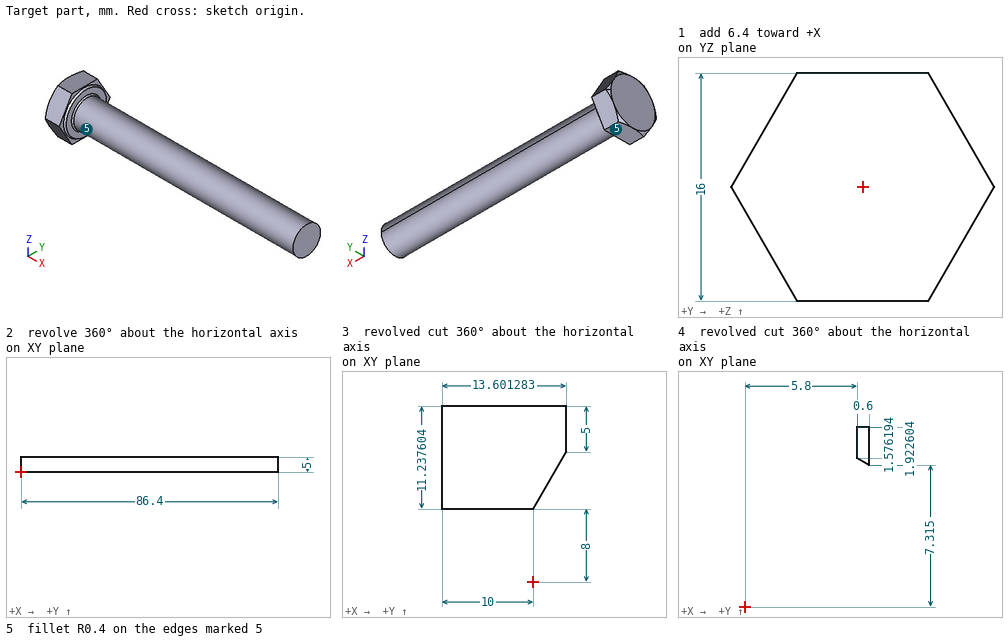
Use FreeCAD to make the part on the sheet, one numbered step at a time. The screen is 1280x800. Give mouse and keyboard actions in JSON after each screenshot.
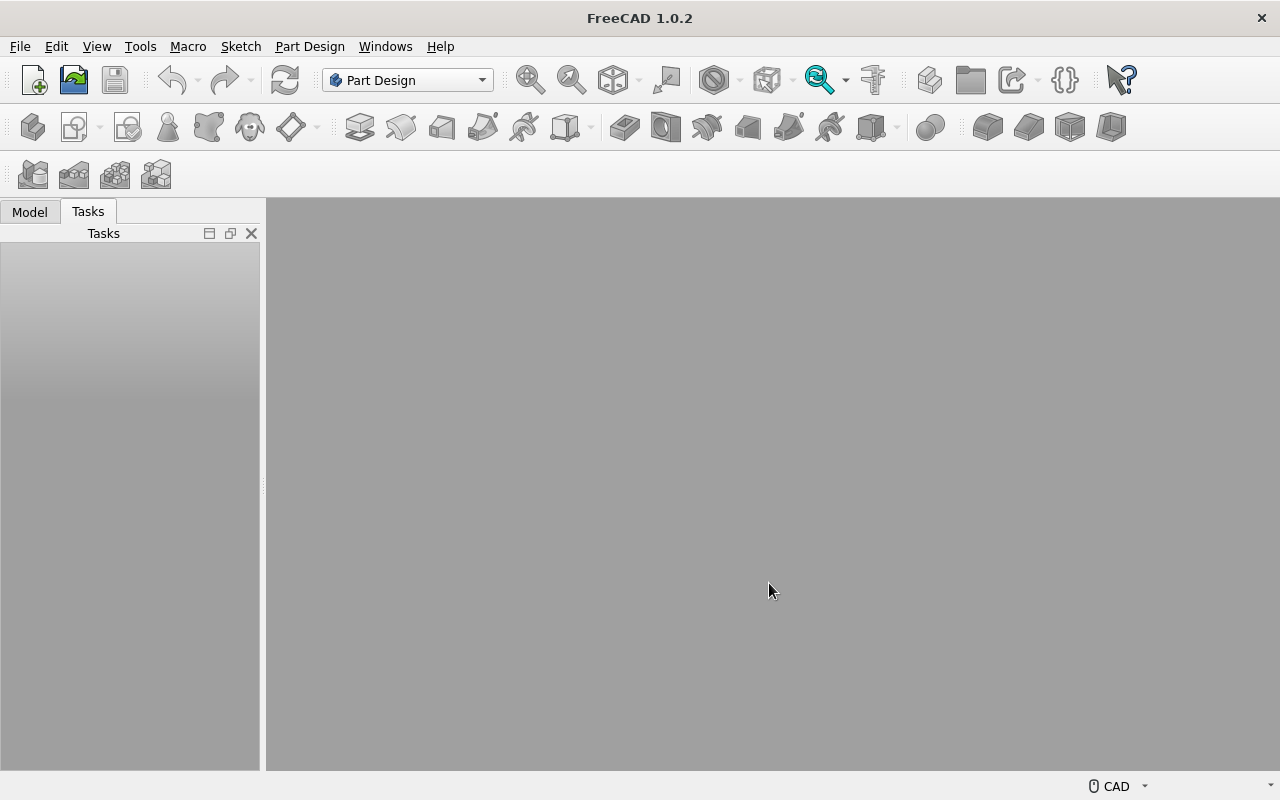
{"action": "left_click", "coordinate": [33, 80]}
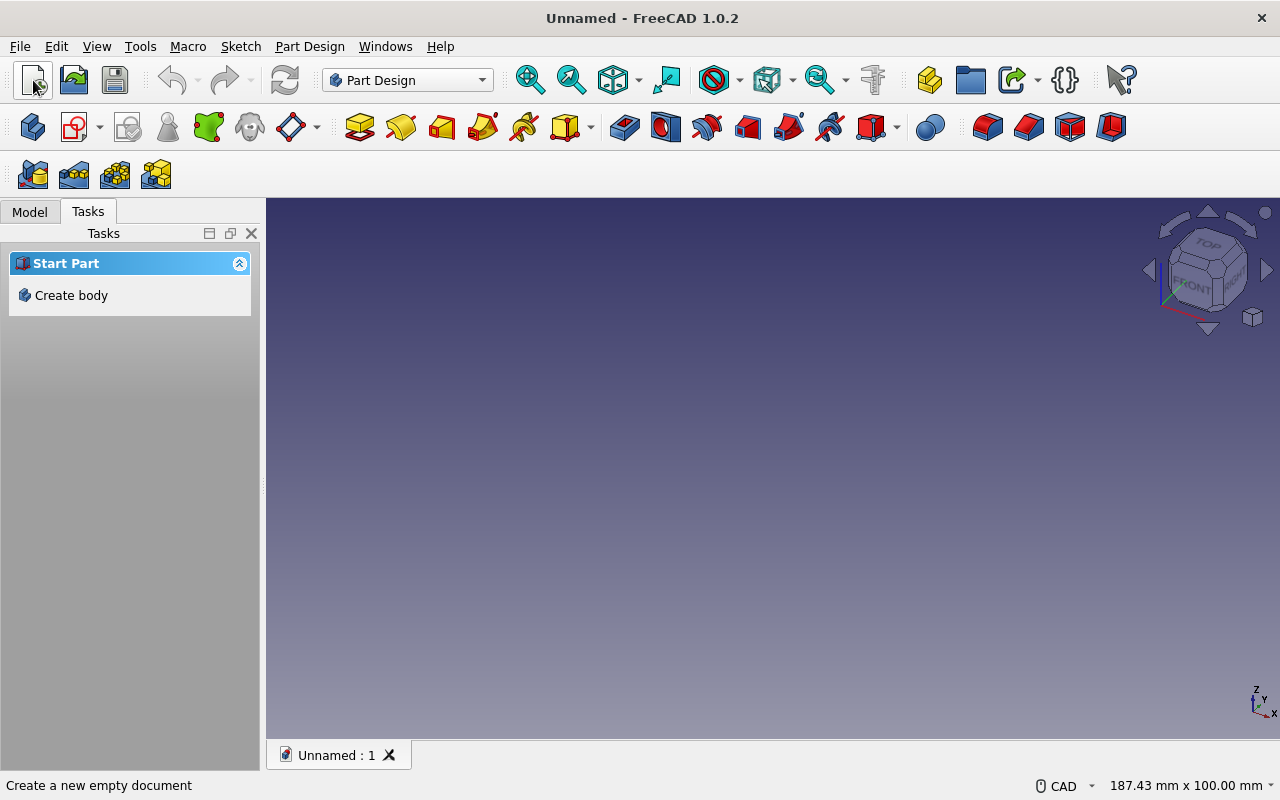
{"action": "left_click", "coordinate": [74, 128]}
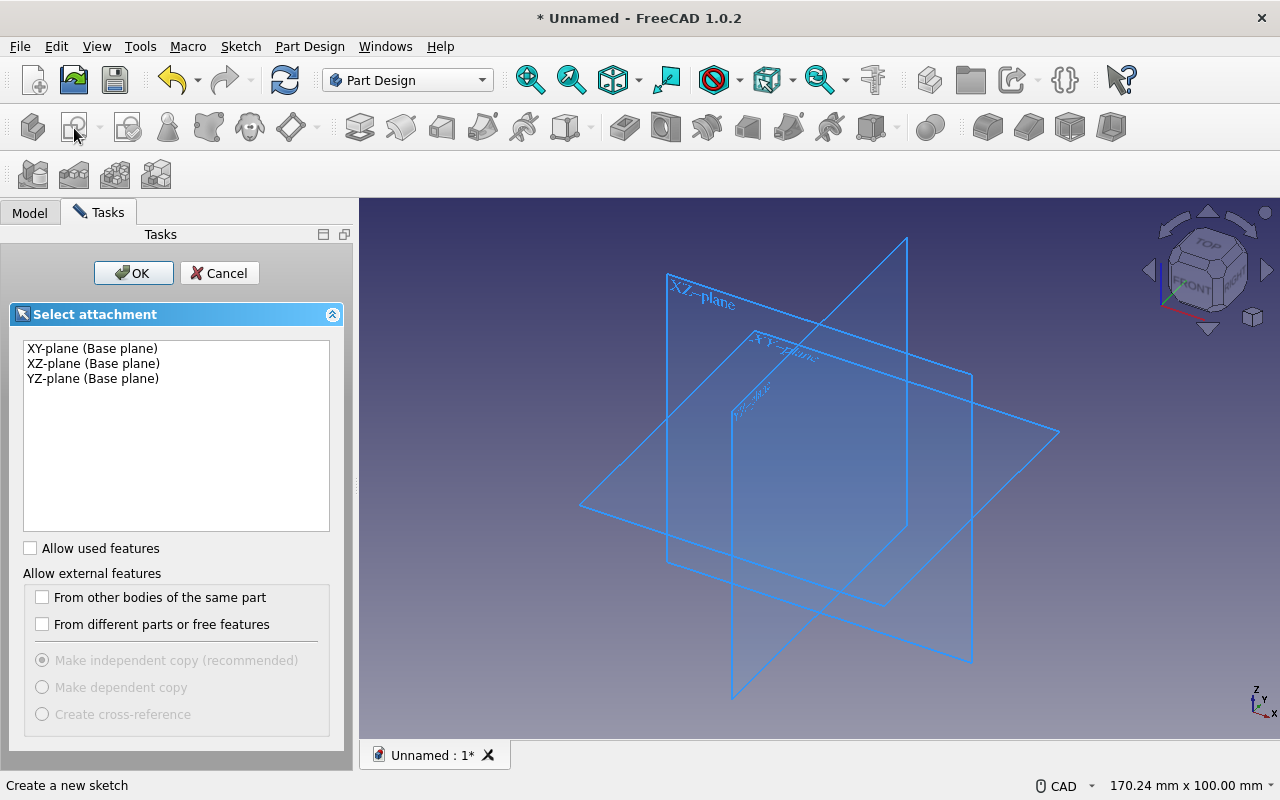
{"action": "left_click", "coordinate": [84, 378]}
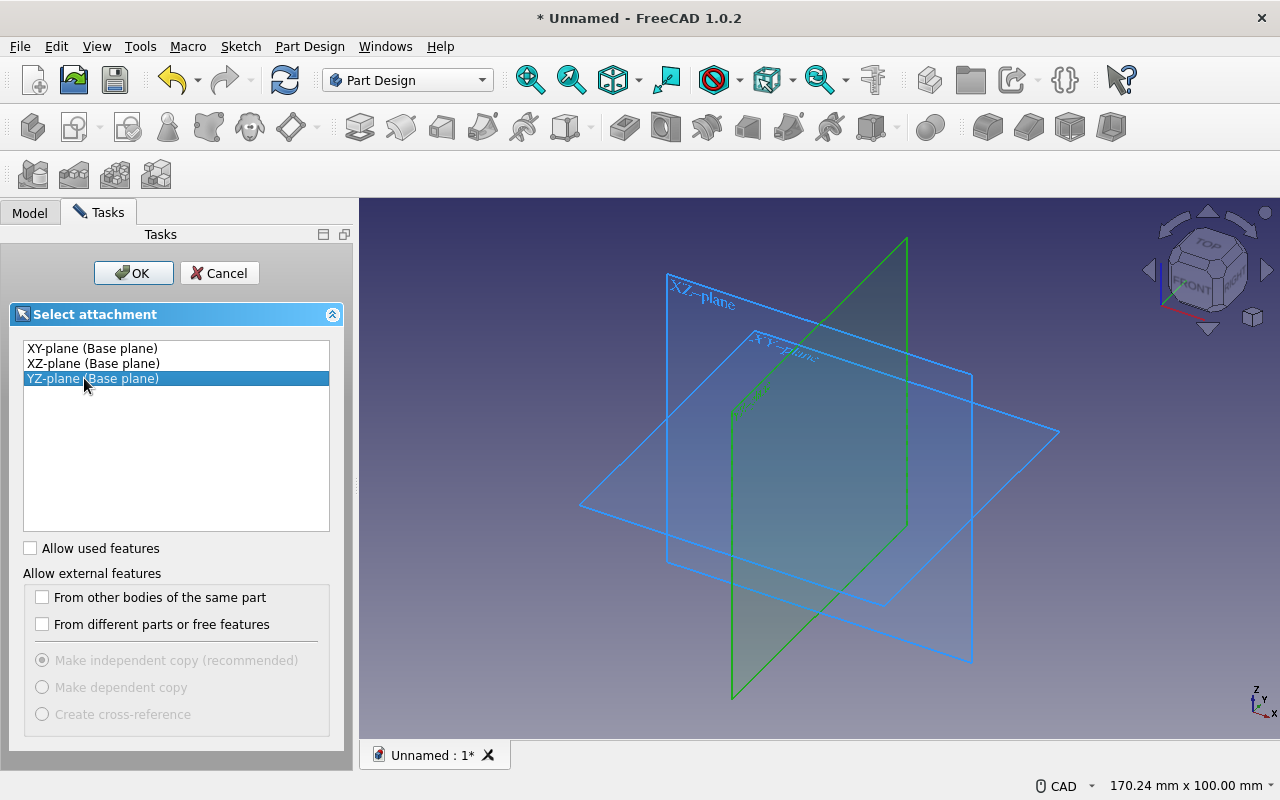
{"action": "left_click", "coordinate": [134, 273]}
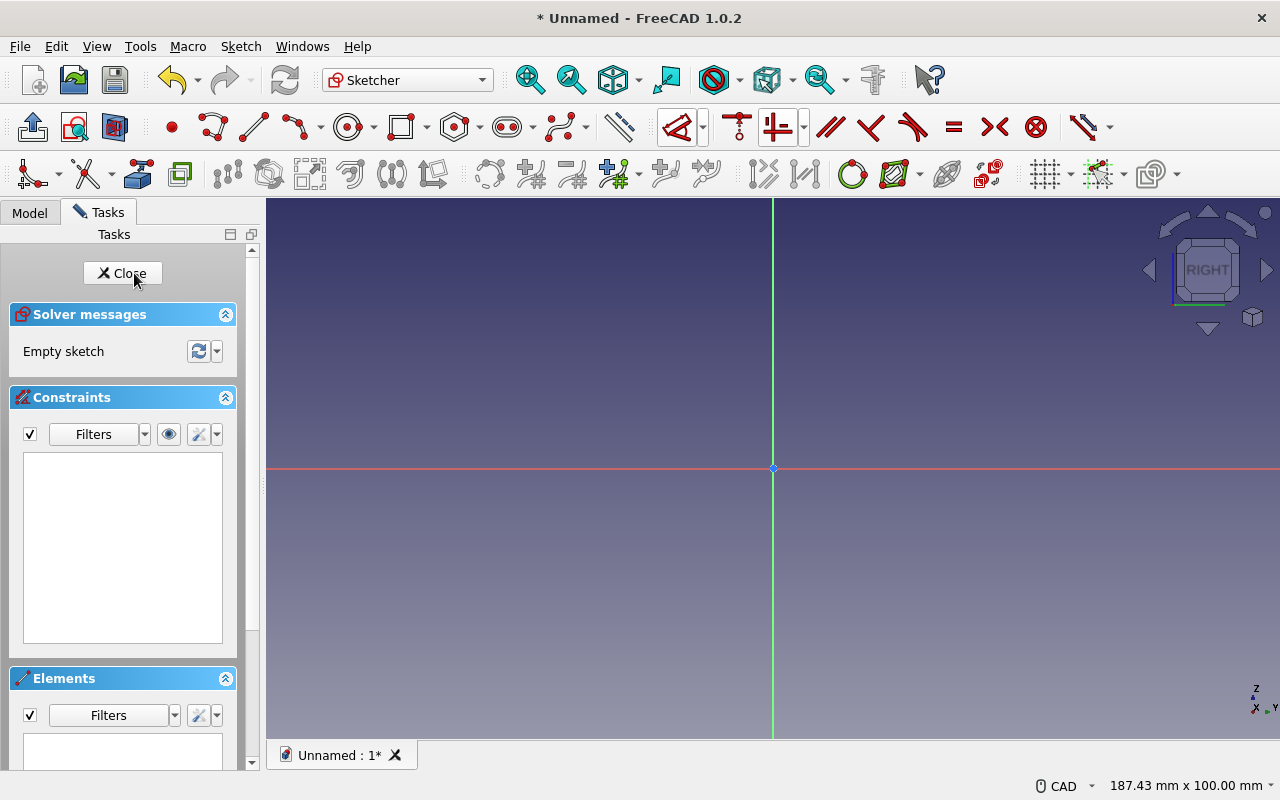
{"action": "scroll", "coordinate": [795, 468], "scroll_direction": "up", "scroll_amount": 7}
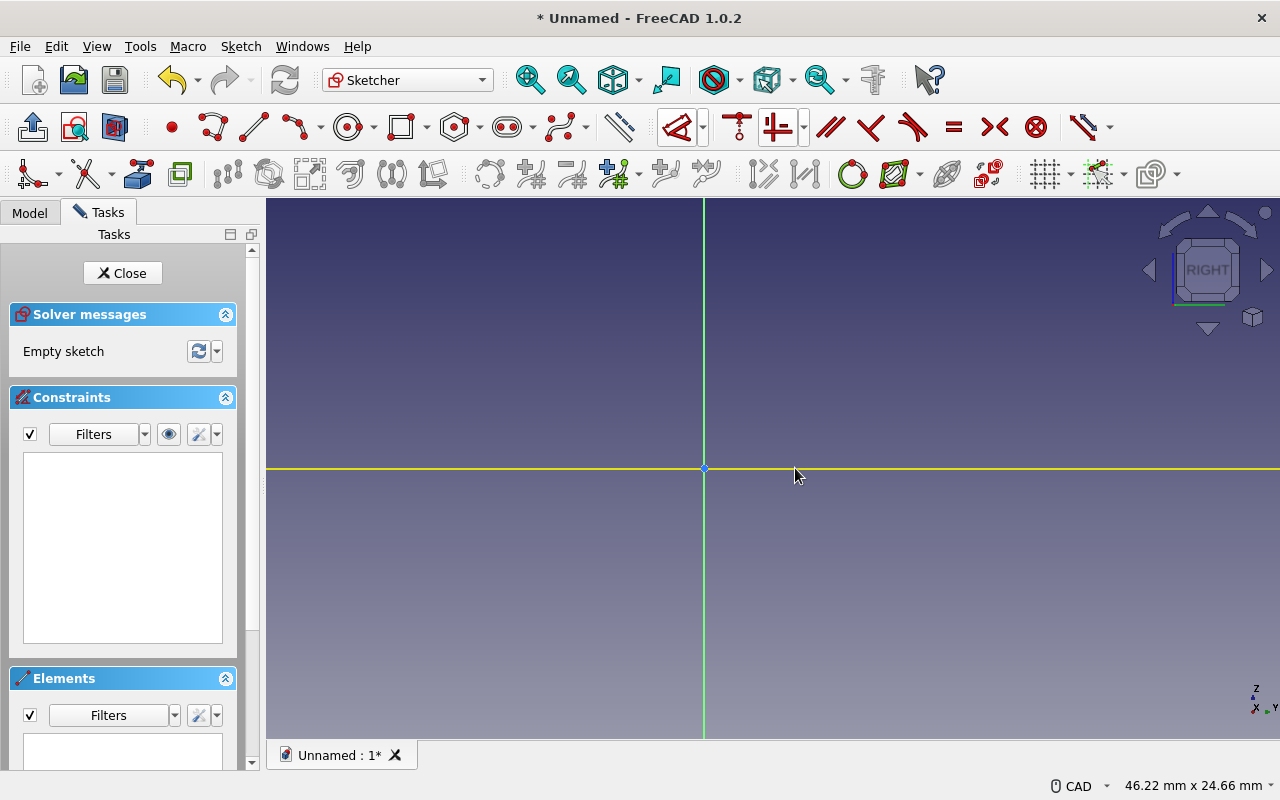
{"action": "left_click", "coordinate": [454, 128]}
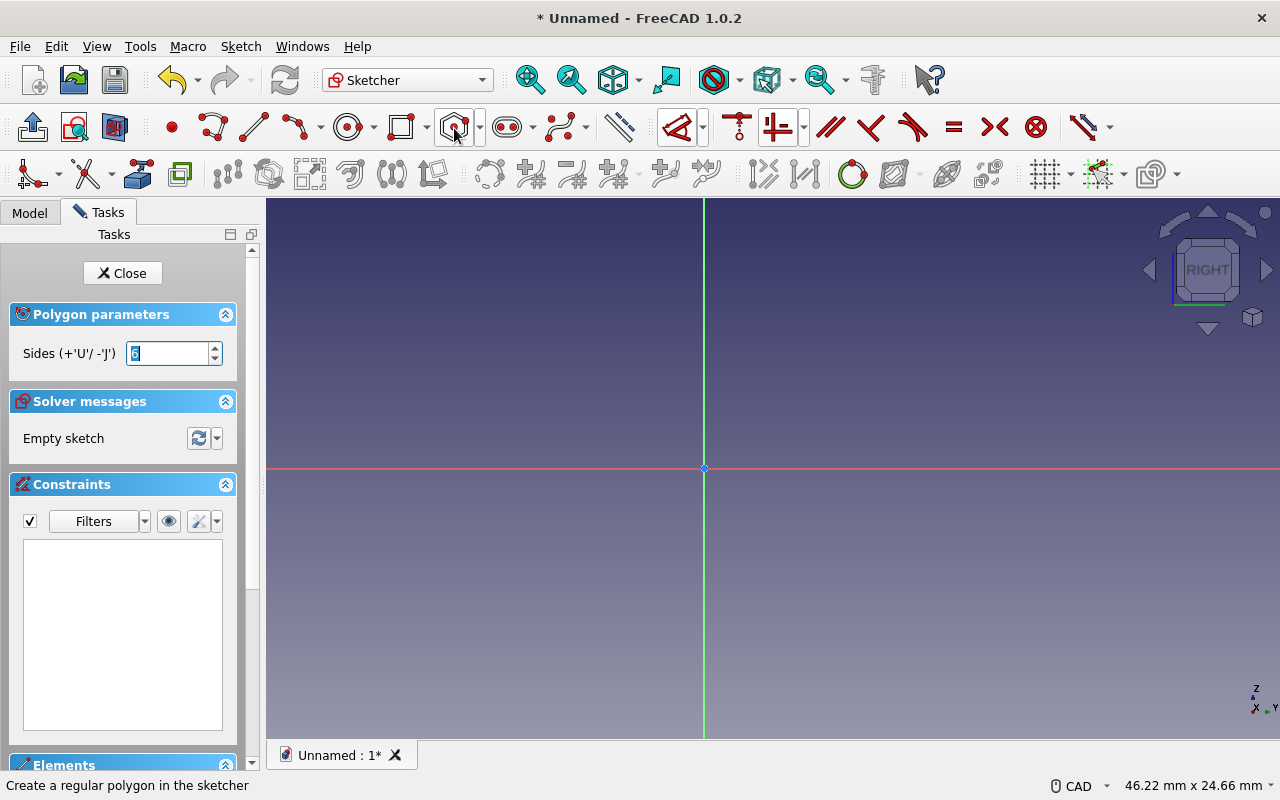
{"action": "left_click", "coordinate": [704, 468]}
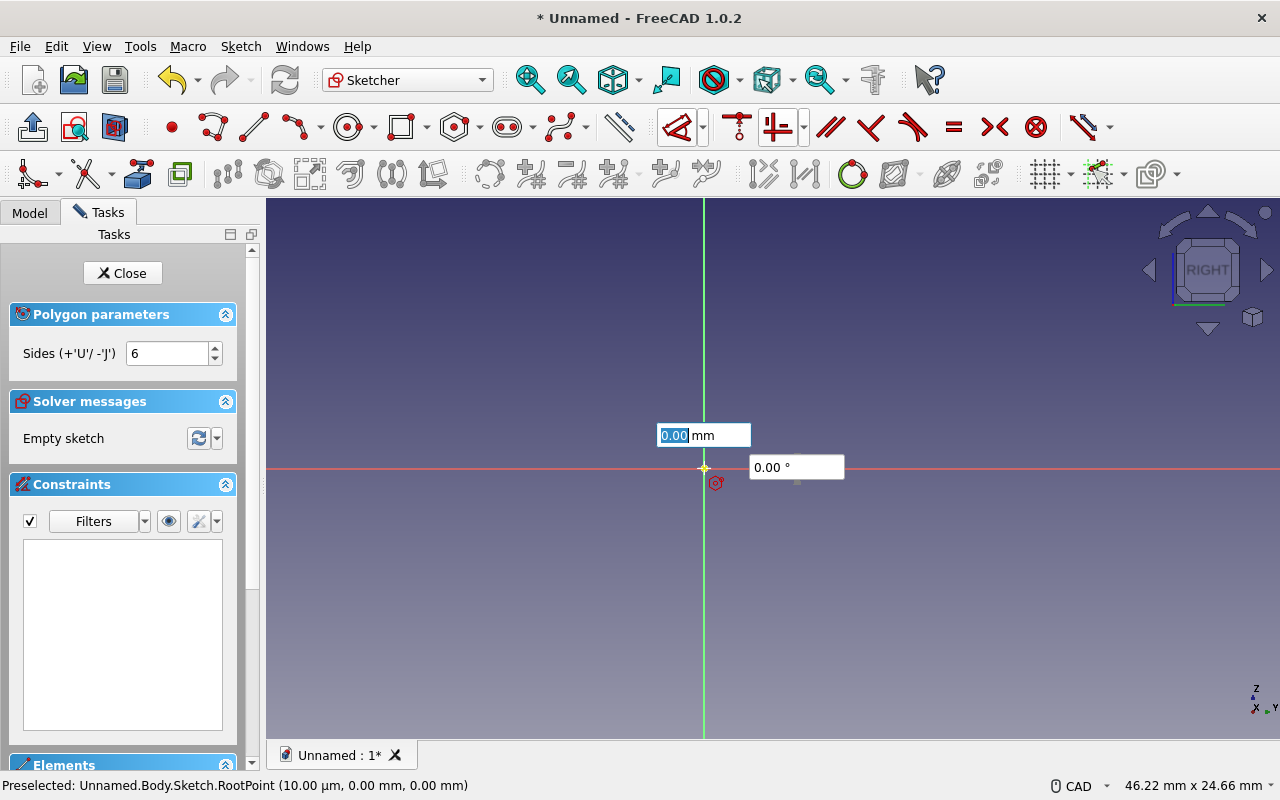
{"action": "left_click", "coordinate": [907, 468]}
{"action": "right_click", "coordinate": [907, 468]}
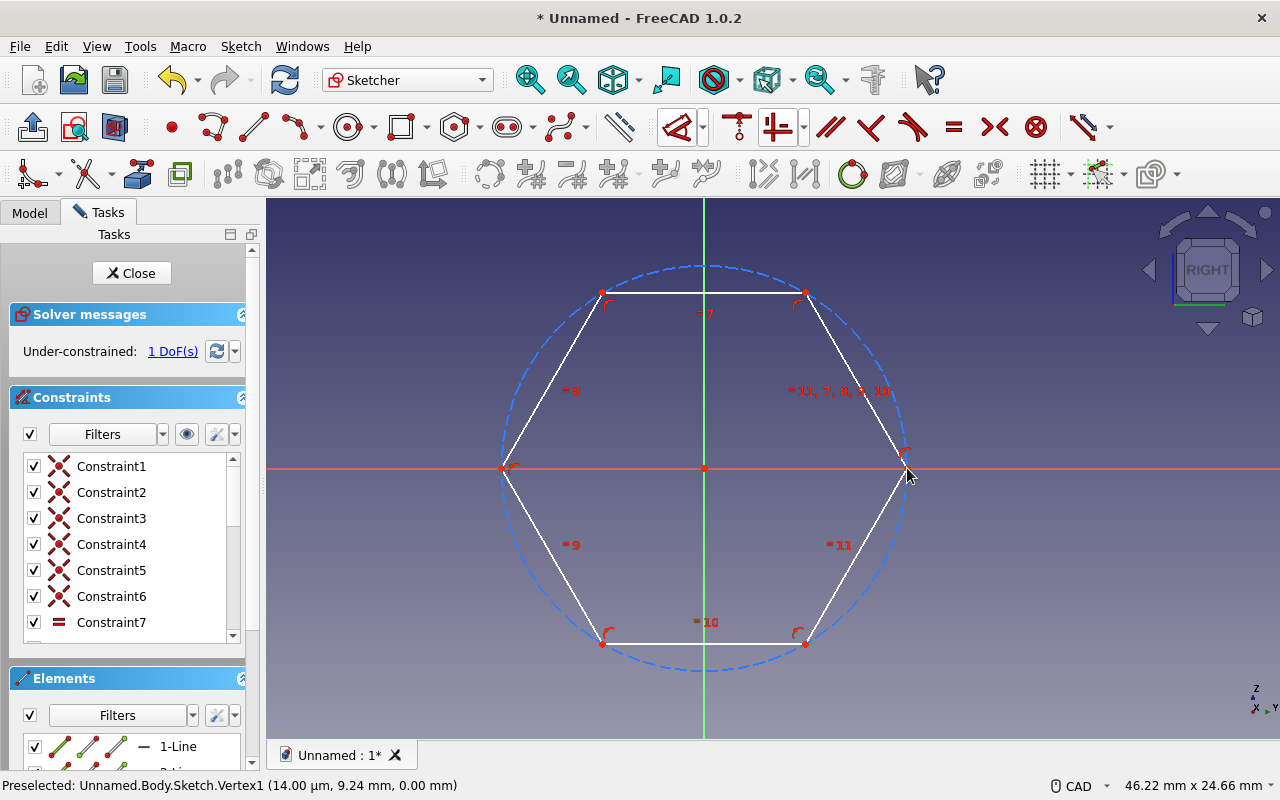
{"action": "left_click", "coordinate": [603, 644]}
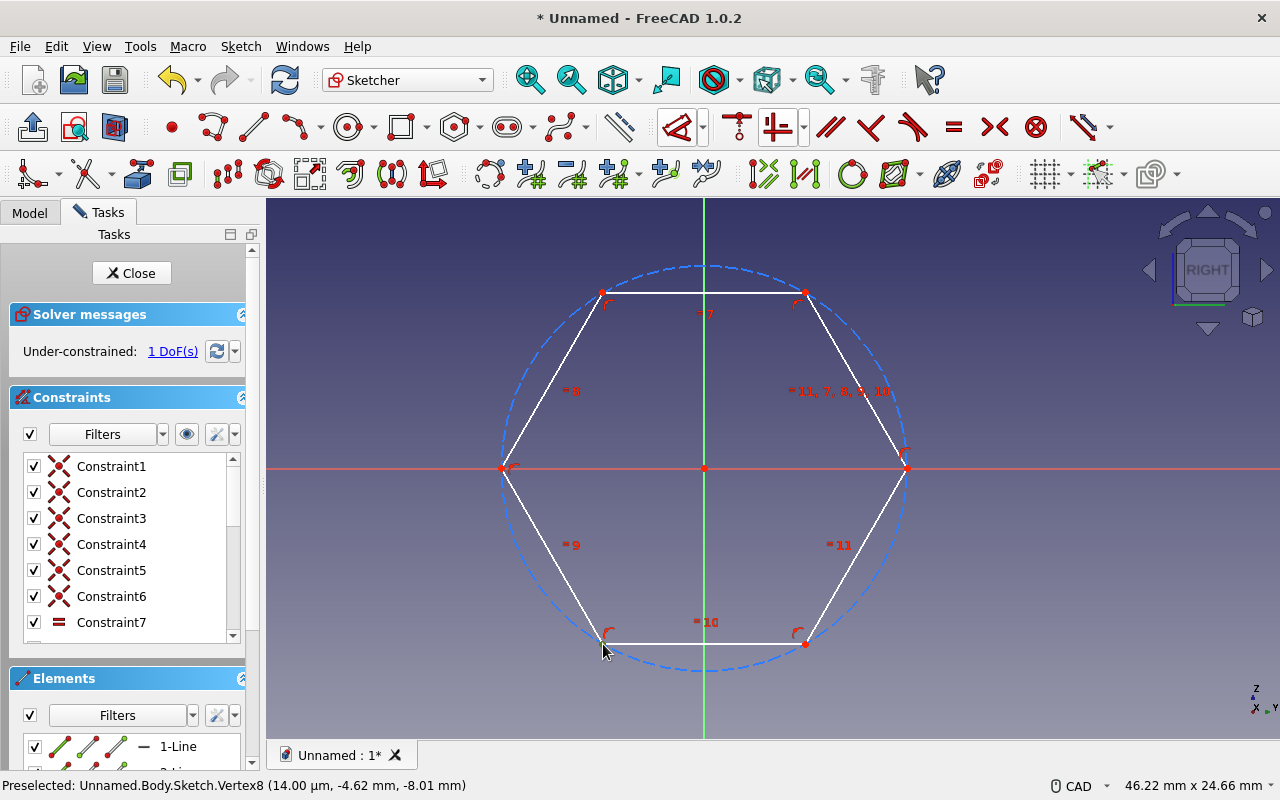
{"action": "left_click", "coordinate": [806, 293]}